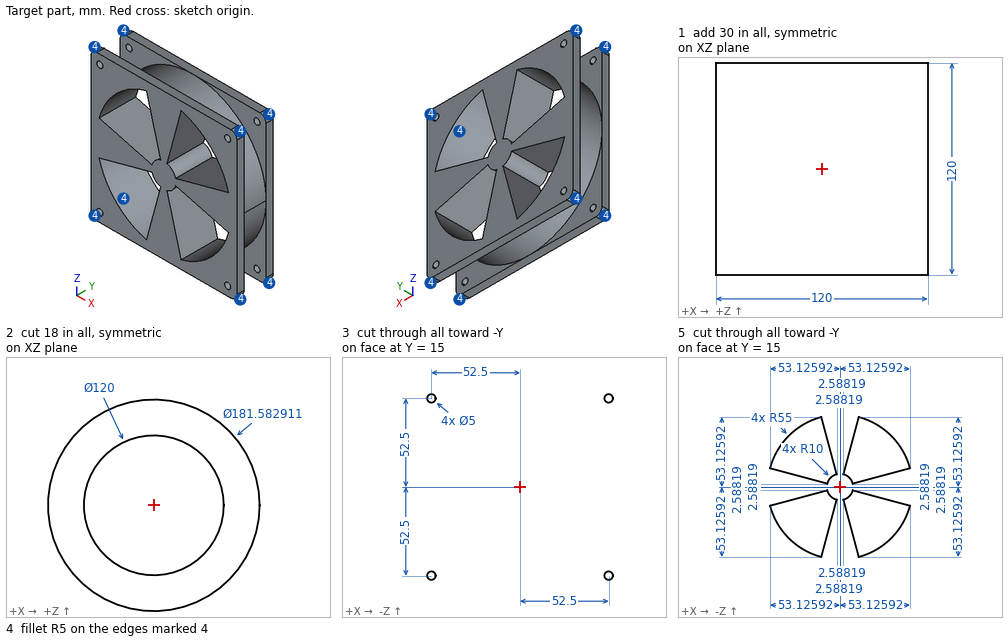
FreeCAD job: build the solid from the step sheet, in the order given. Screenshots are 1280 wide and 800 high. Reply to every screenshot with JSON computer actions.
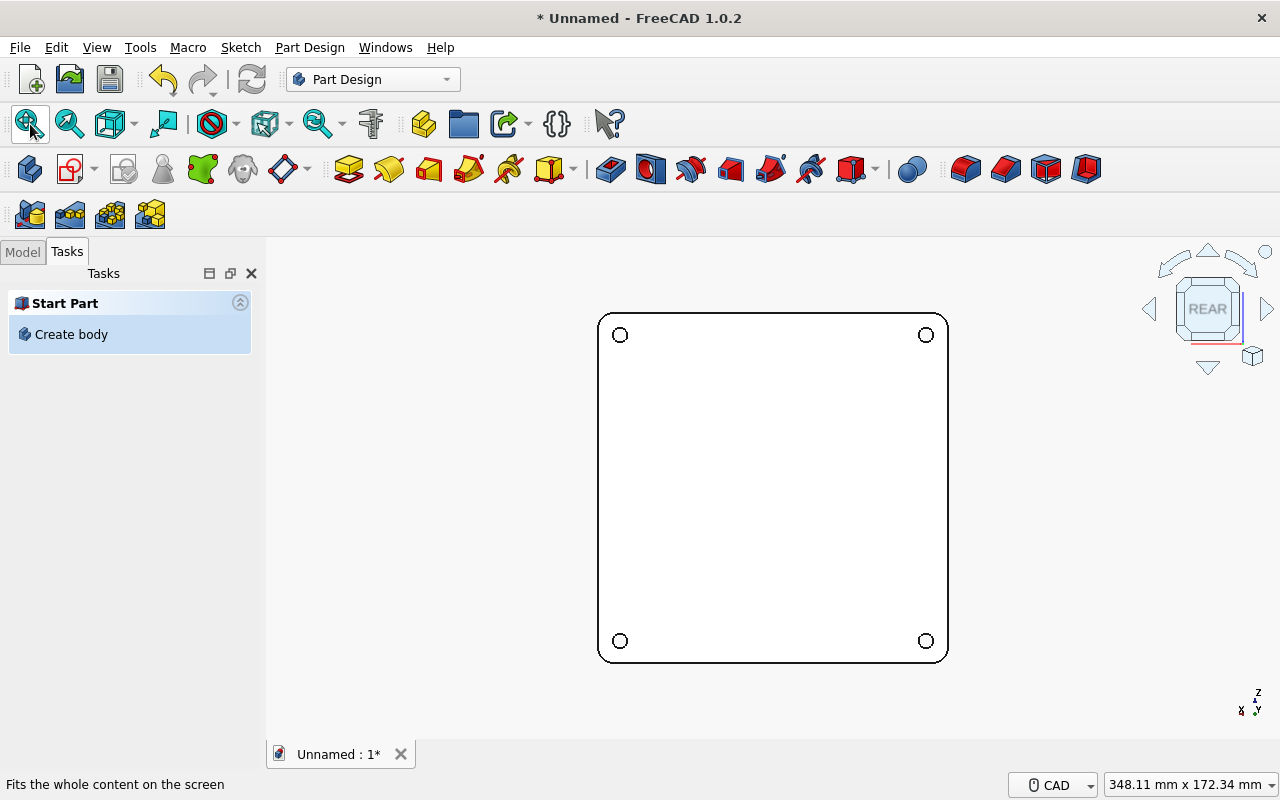
{"action": "left_click", "coordinate": [773, 487]}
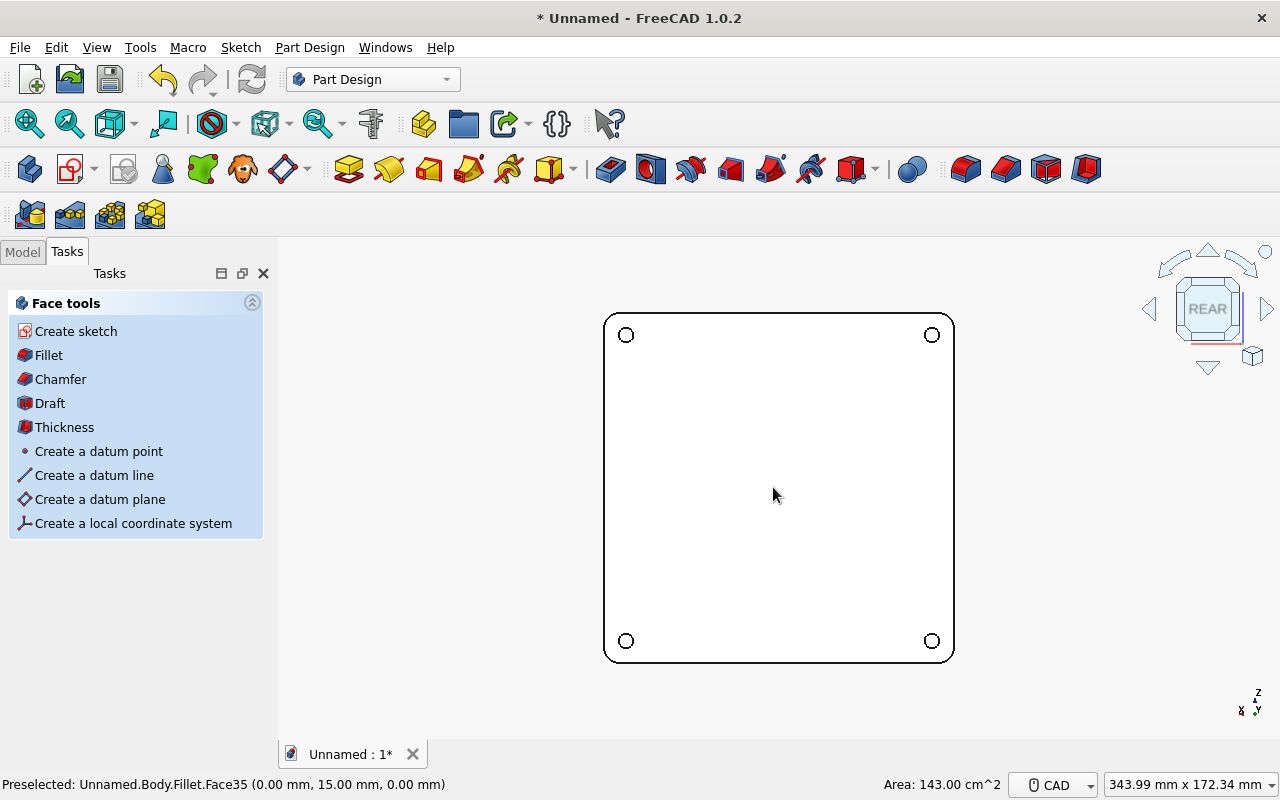
{"action": "left_click", "coordinate": [70, 170]}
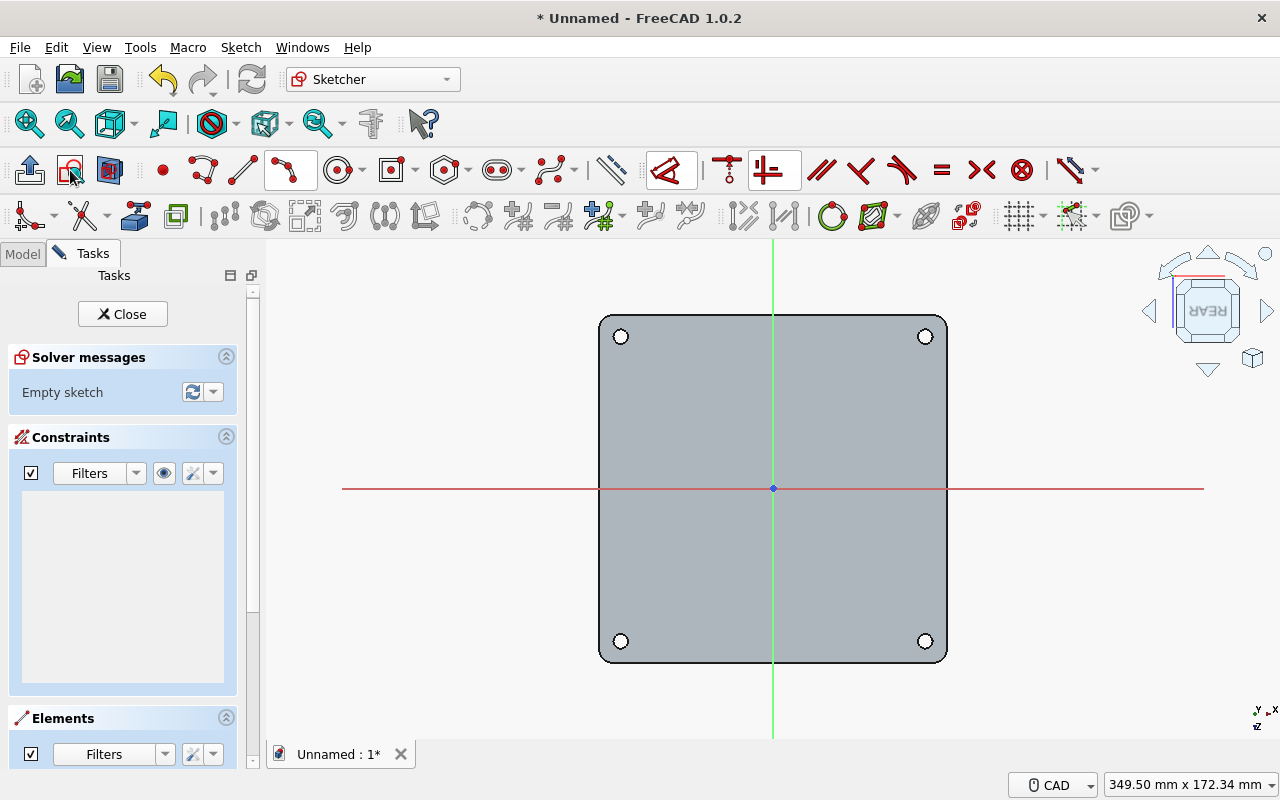
{"action": "left_click", "coordinate": [244, 170]}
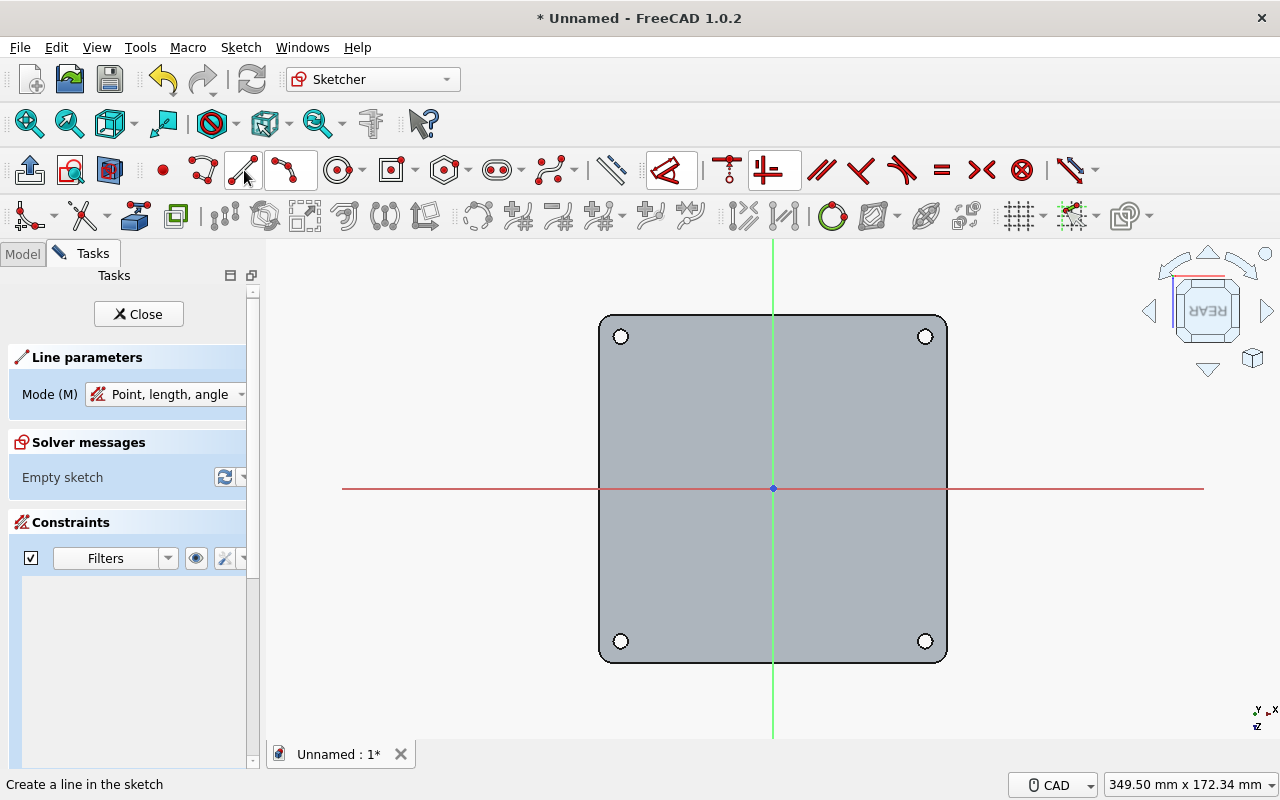
{"action": "scroll", "coordinate": [765, 461], "scroll_direction": "up", "scroll_amount": 4}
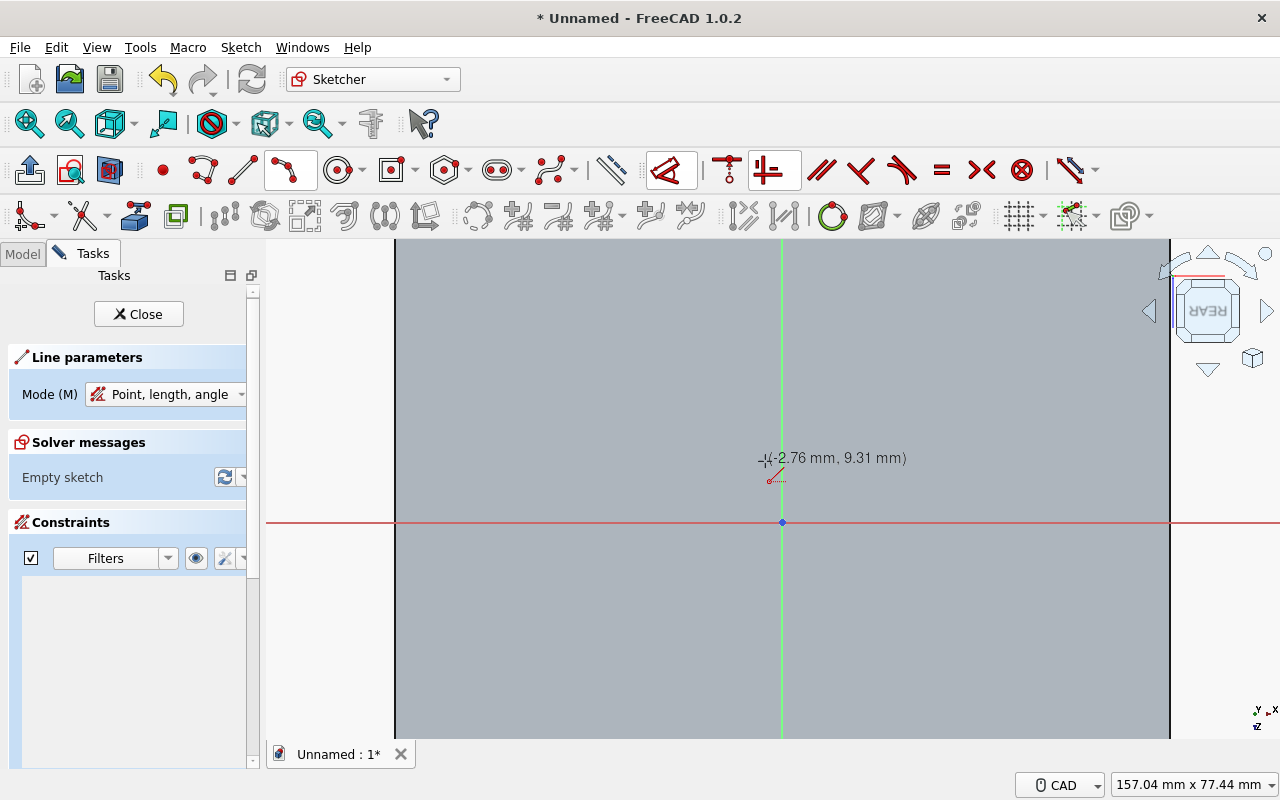
{"action": "left_click", "coordinate": [765, 460]}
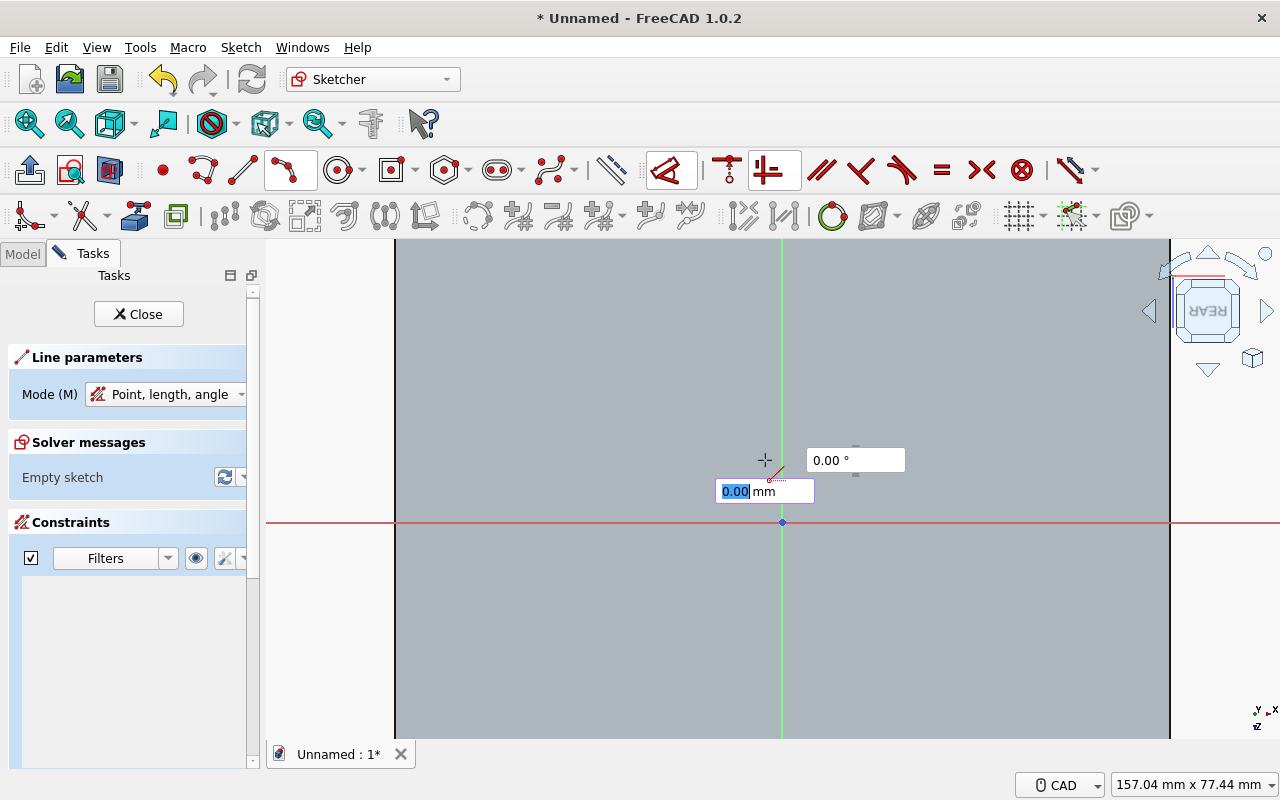
{"action": "scroll", "coordinate": [641, 461], "scroll_direction": "down", "scroll_amount": 4}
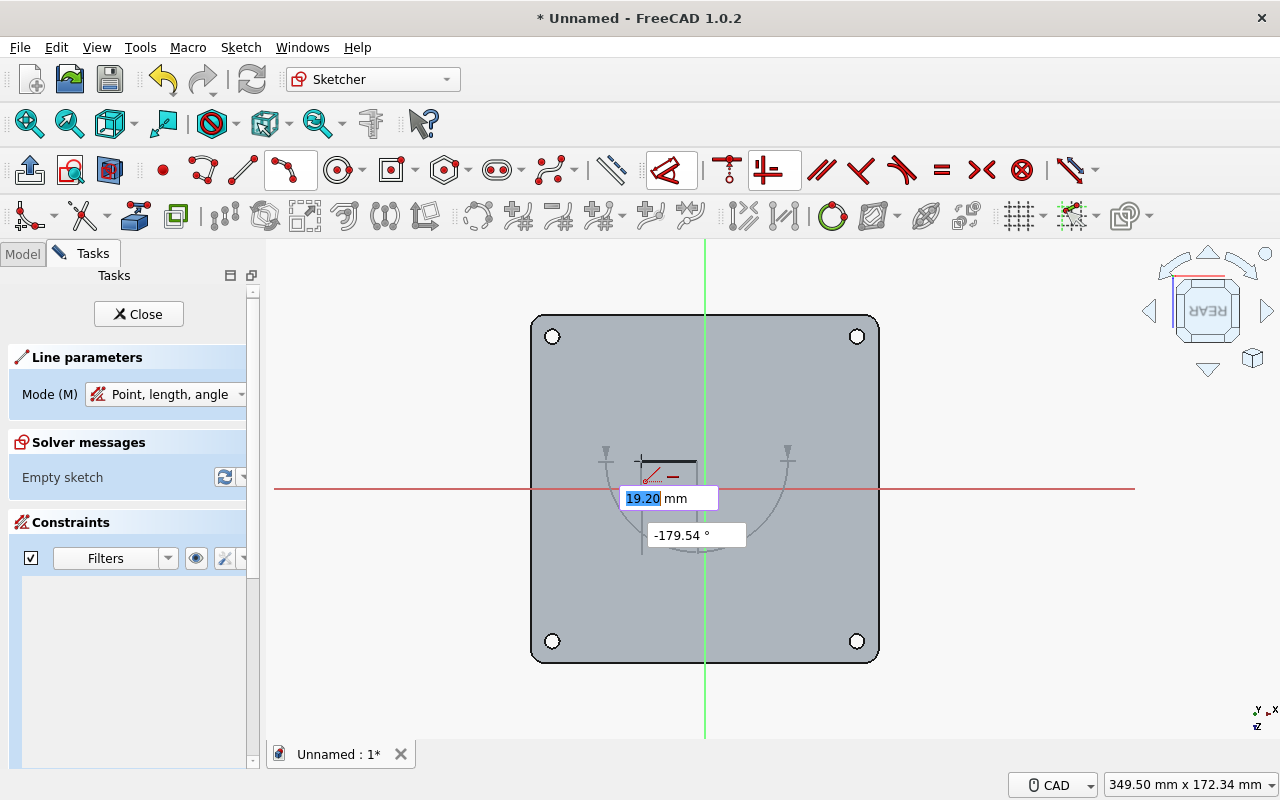
{"action": "left_click", "coordinate": [663, 335]}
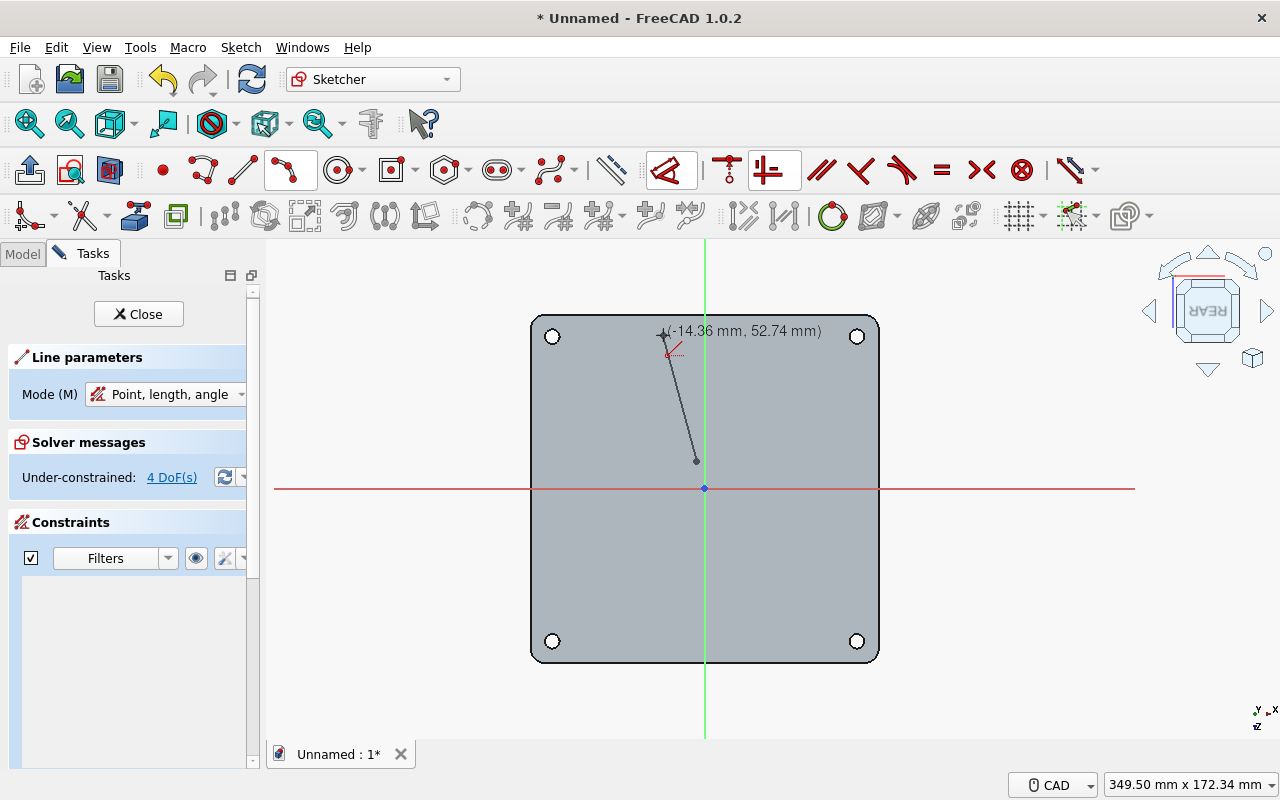
{"action": "left_click", "coordinate": [551, 448]}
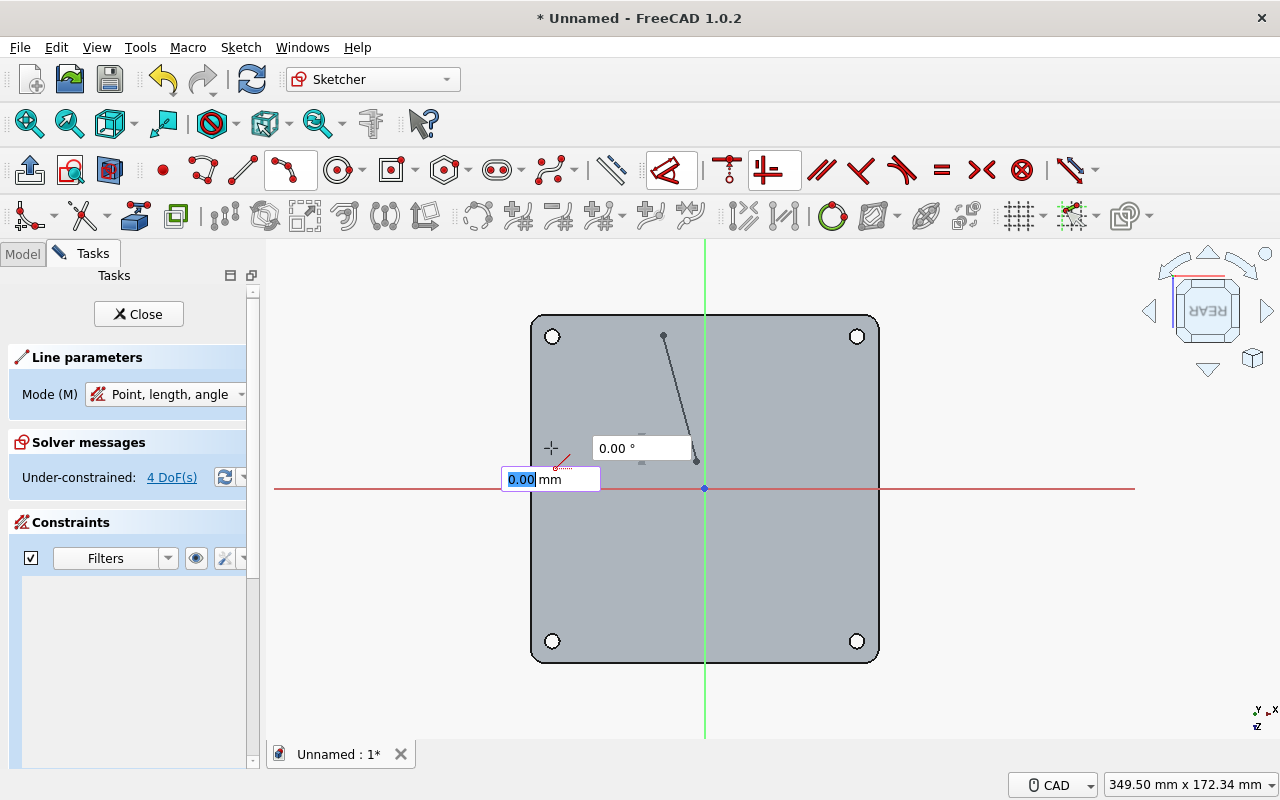
{"action": "scroll", "coordinate": [677, 481], "scroll_direction": "up", "scroll_amount": 4}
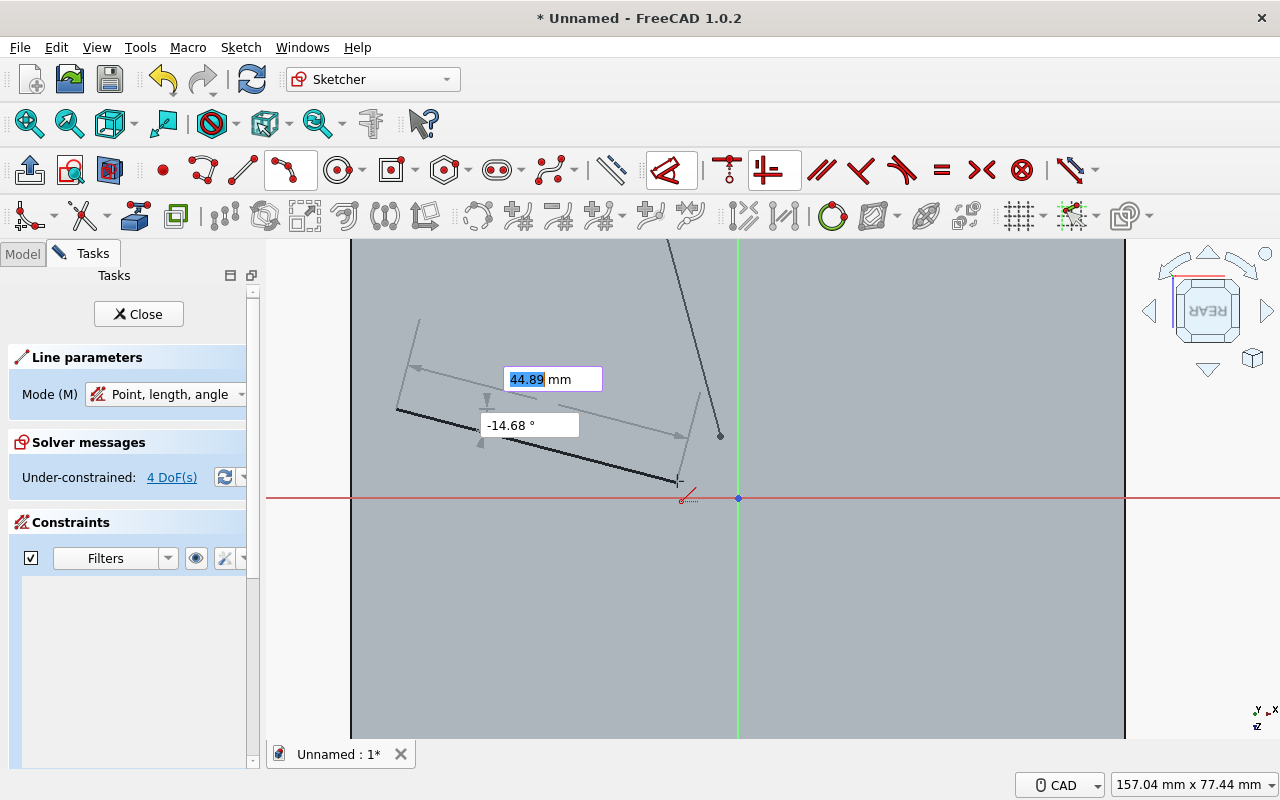
{"action": "left_click", "coordinate": [676, 481]}